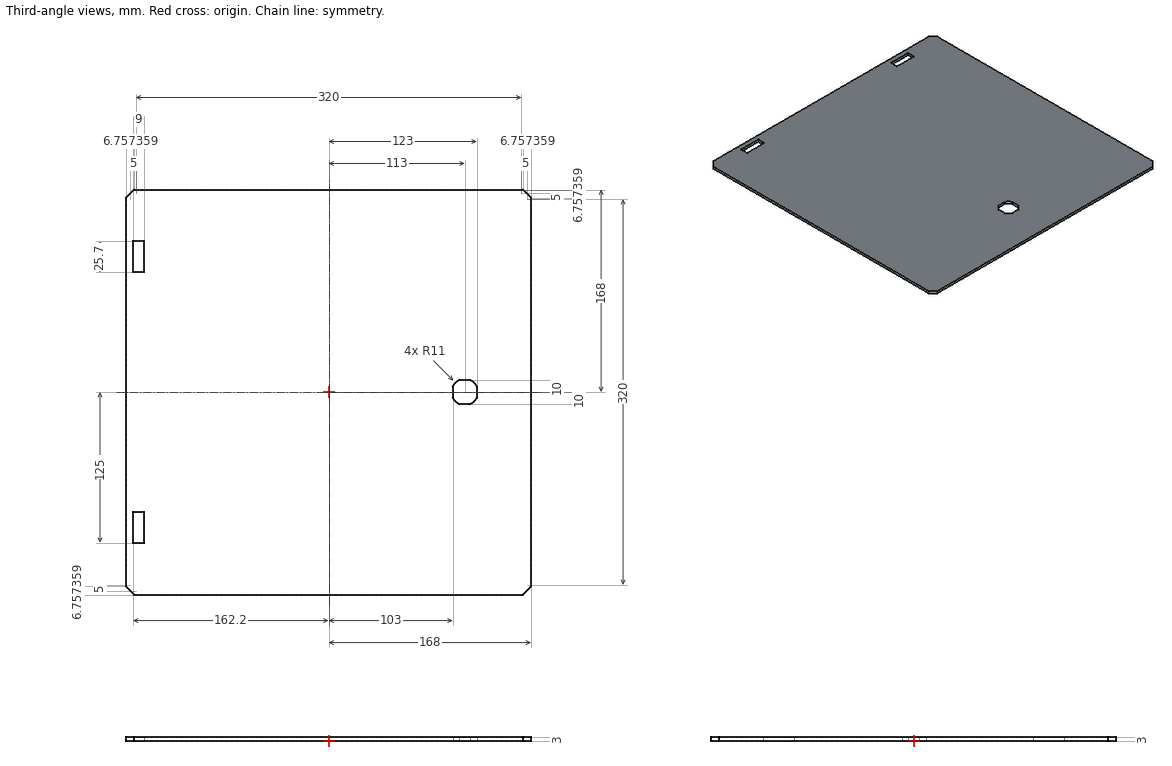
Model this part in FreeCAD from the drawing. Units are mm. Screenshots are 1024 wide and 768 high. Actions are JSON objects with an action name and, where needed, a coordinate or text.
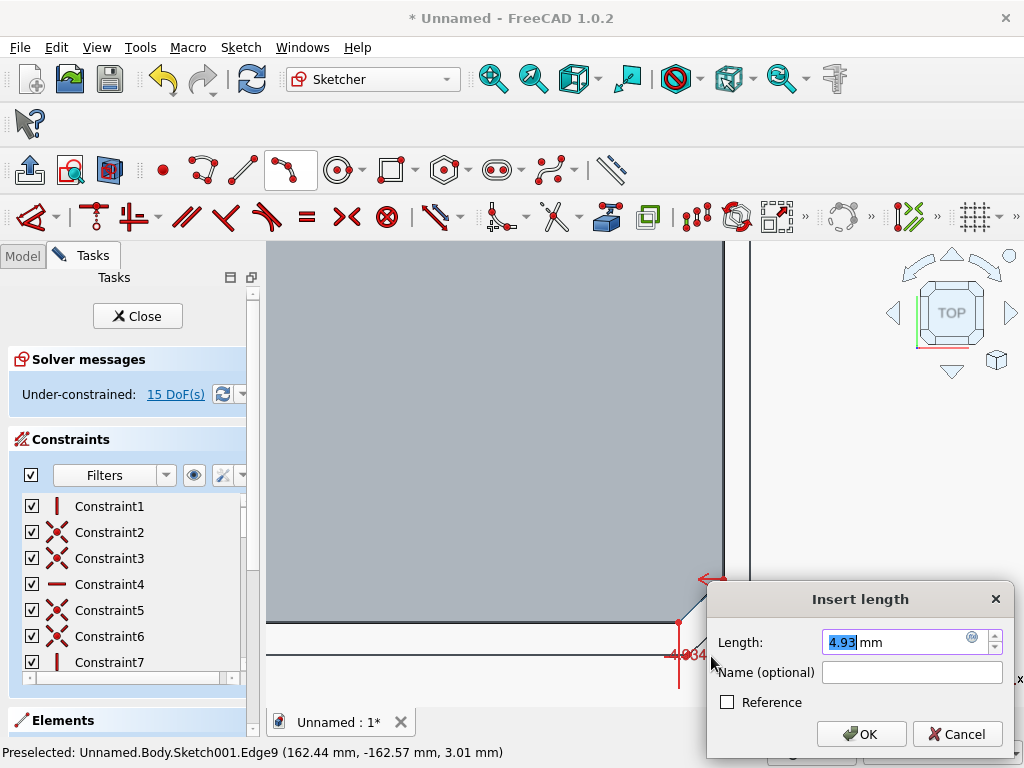
{"action": "type", "text": "5"}
{"action": "key", "text": "Return"}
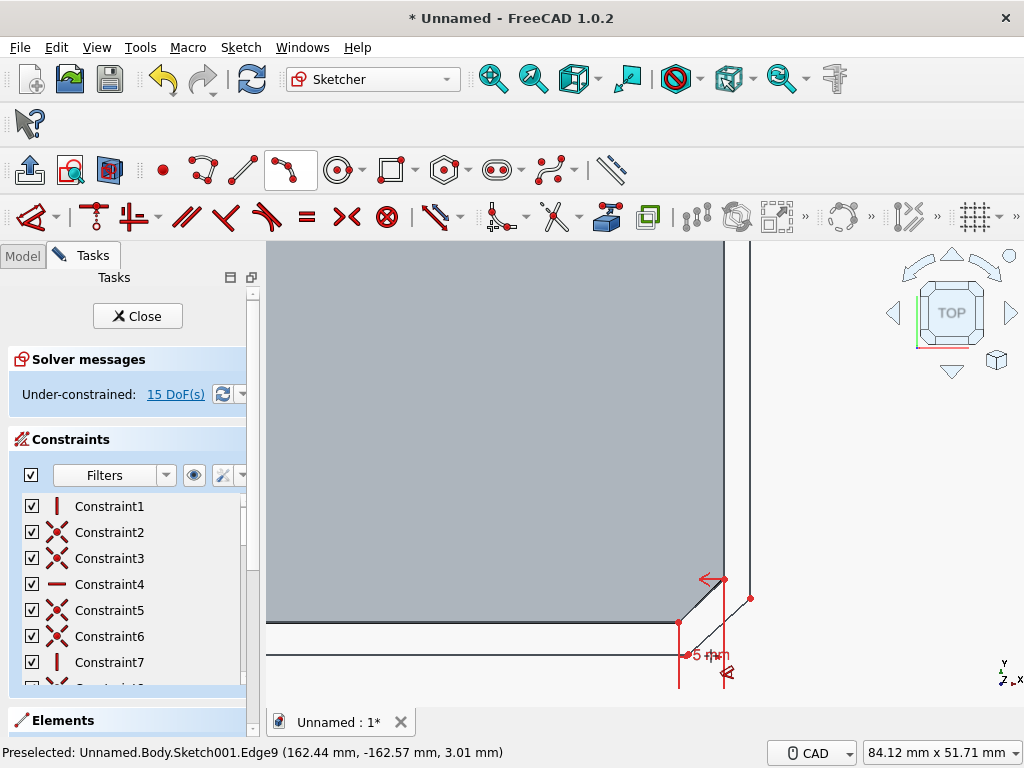
{"action": "left_click", "coordinate": [711, 592]}
{"action": "left_click", "coordinate": [758, 611]}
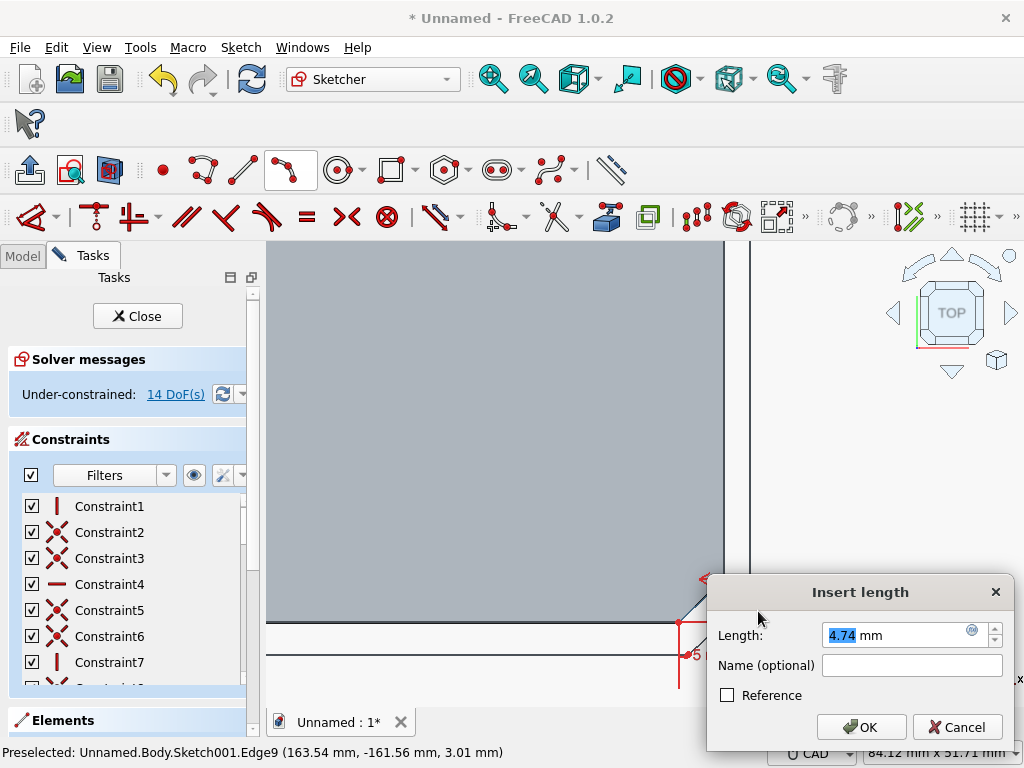
{"action": "type", "text": "5"}
{"action": "key", "text": "Return"}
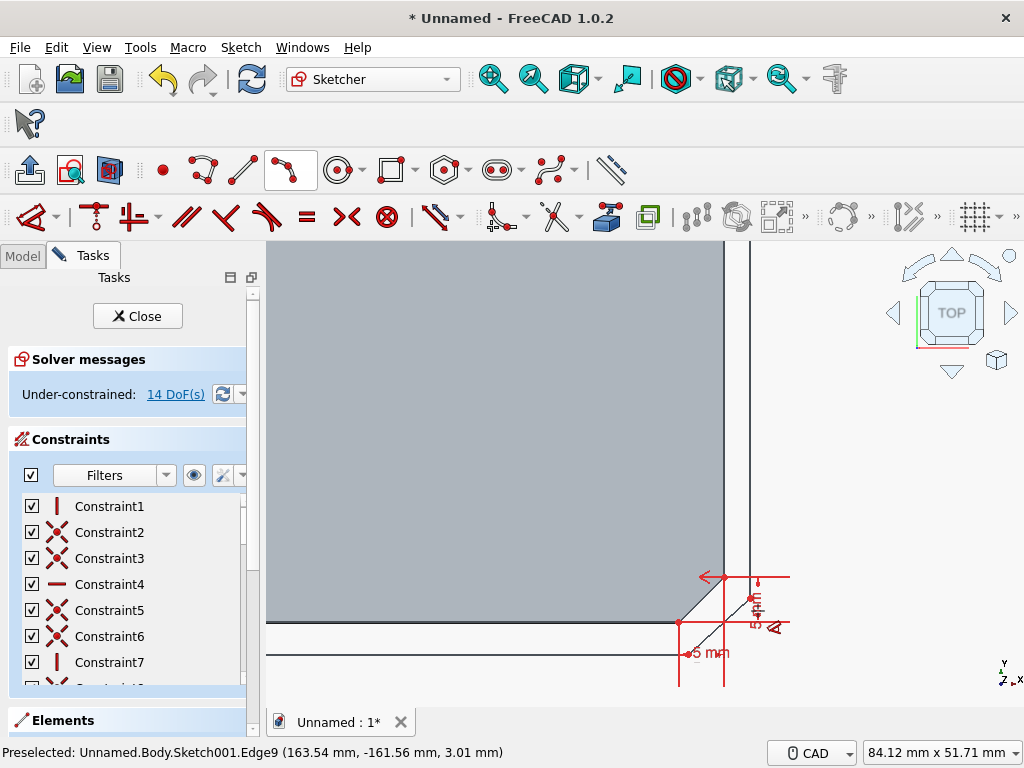
{"action": "scroll", "coordinate": [710, 607], "scroll_direction": "down", "scroll_amount": 12}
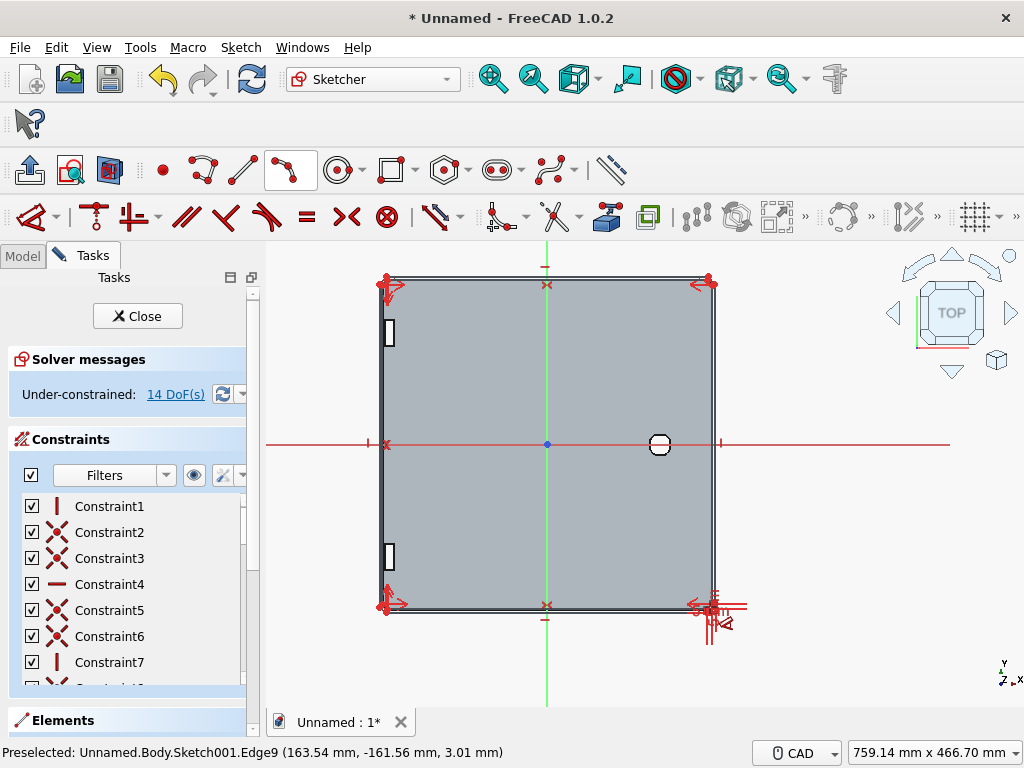
{"action": "scroll", "coordinate": [445, 608], "scroll_direction": "up", "scroll_amount": 12}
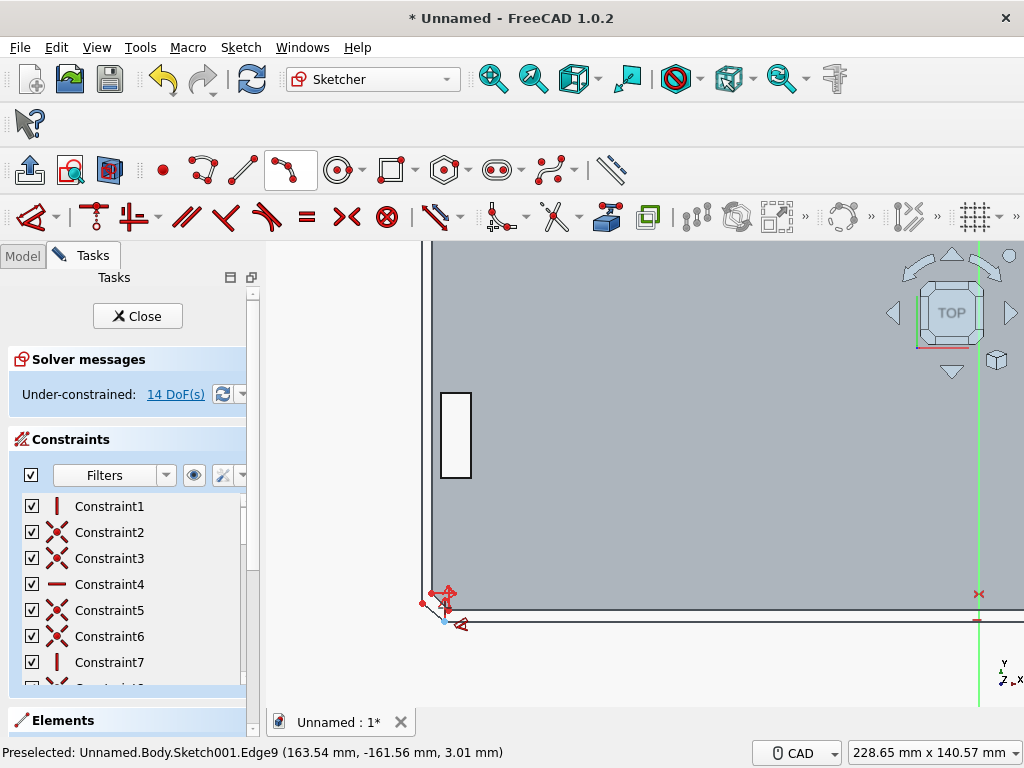
{"action": "left_click", "coordinate": [441, 599]}
{"action": "left_click", "coordinate": [421, 646]}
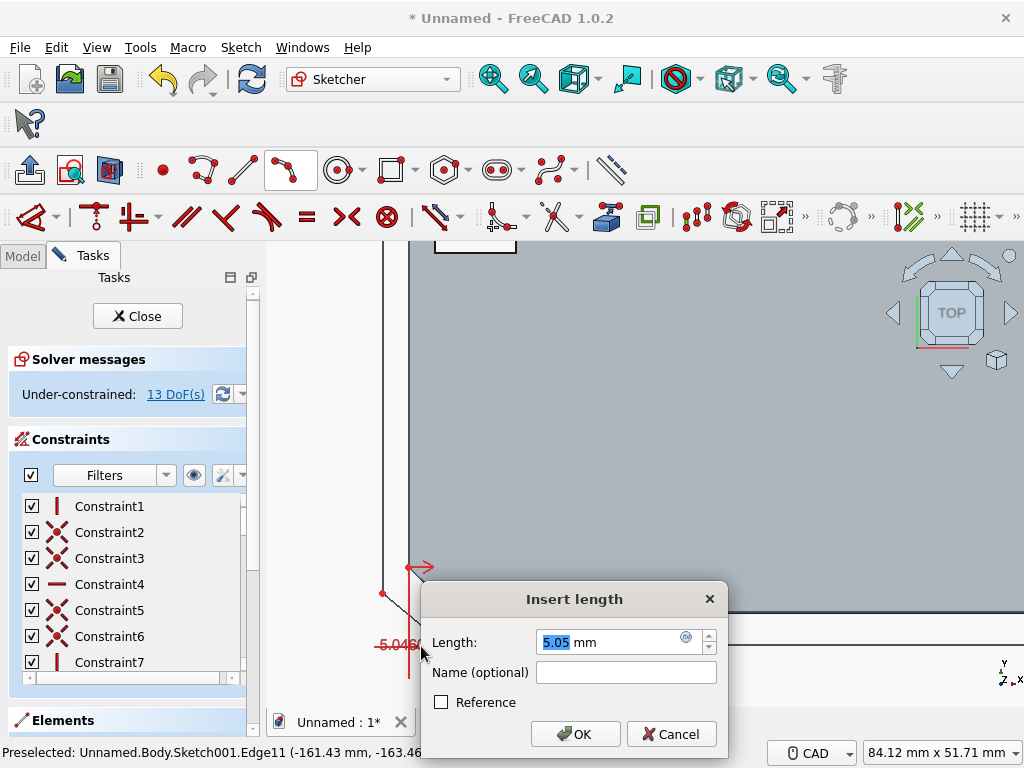
{"action": "type", "text": "5"}
{"action": "key", "text": "Return"}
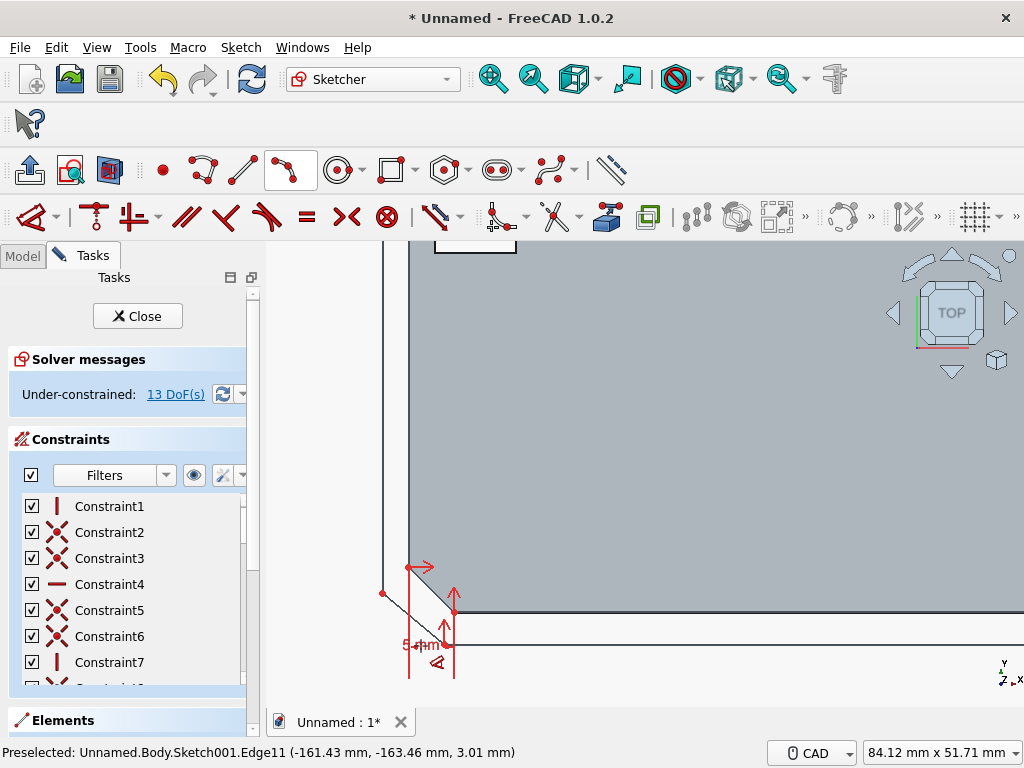
{"action": "scroll", "coordinate": [445, 608], "scroll_direction": "down", "scroll_amount": 12}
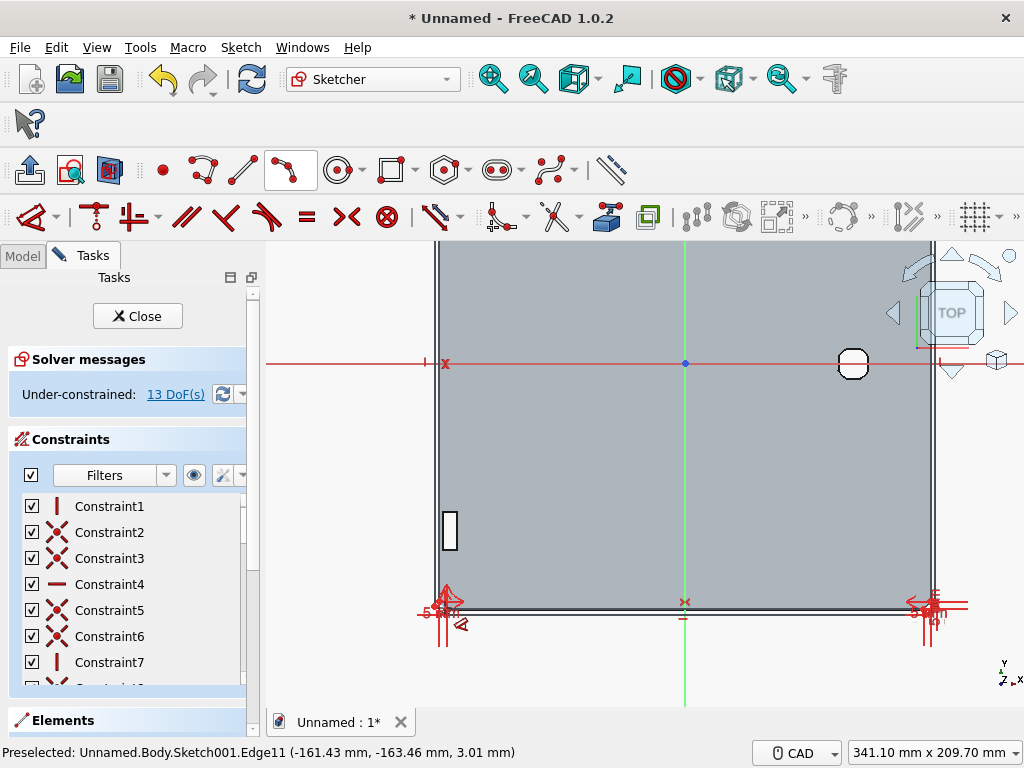
{"action": "scroll", "coordinate": [443, 342], "scroll_direction": "up", "scroll_amount": 12}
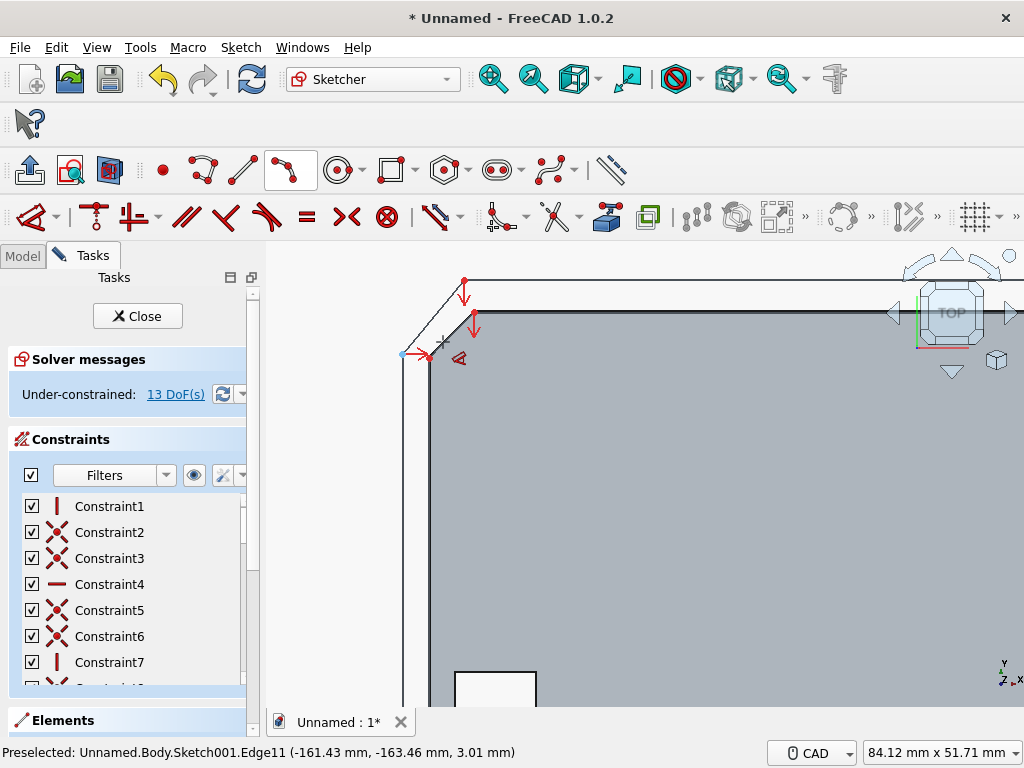
{"action": "left_click", "coordinate": [443, 344]}
{"action": "left_click", "coordinate": [395, 335]}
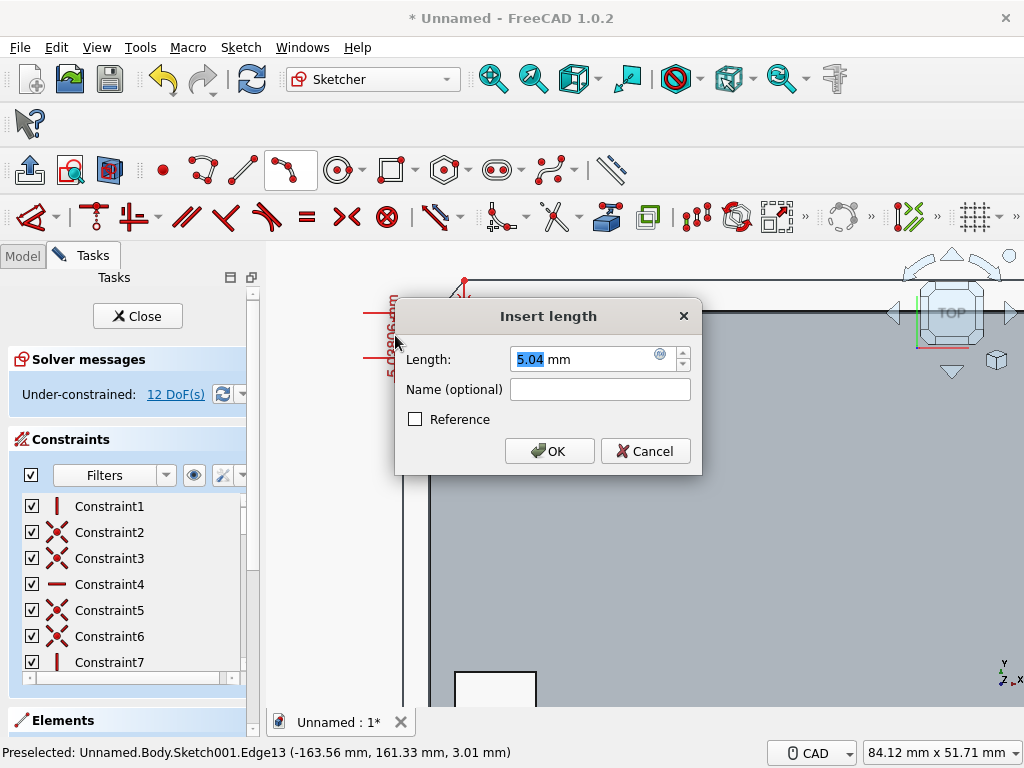
{"action": "type", "text": "5"}
{"action": "key", "text": "Return"}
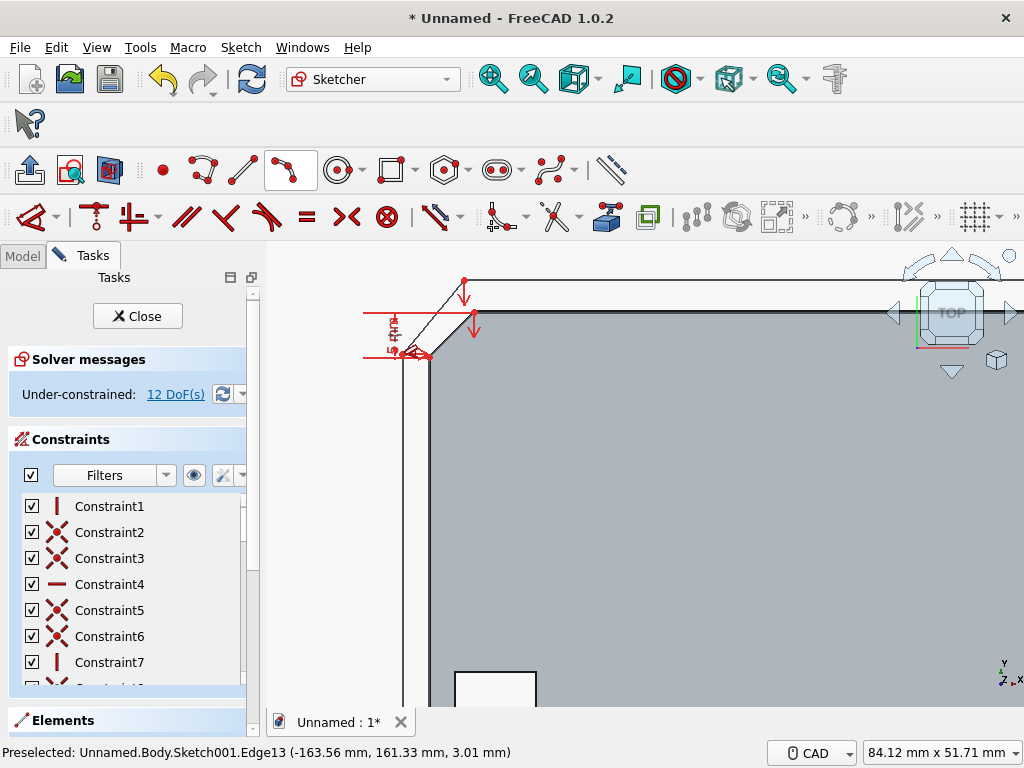
{"action": "scroll", "coordinate": [443, 342], "scroll_direction": "down", "scroll_amount": 12}